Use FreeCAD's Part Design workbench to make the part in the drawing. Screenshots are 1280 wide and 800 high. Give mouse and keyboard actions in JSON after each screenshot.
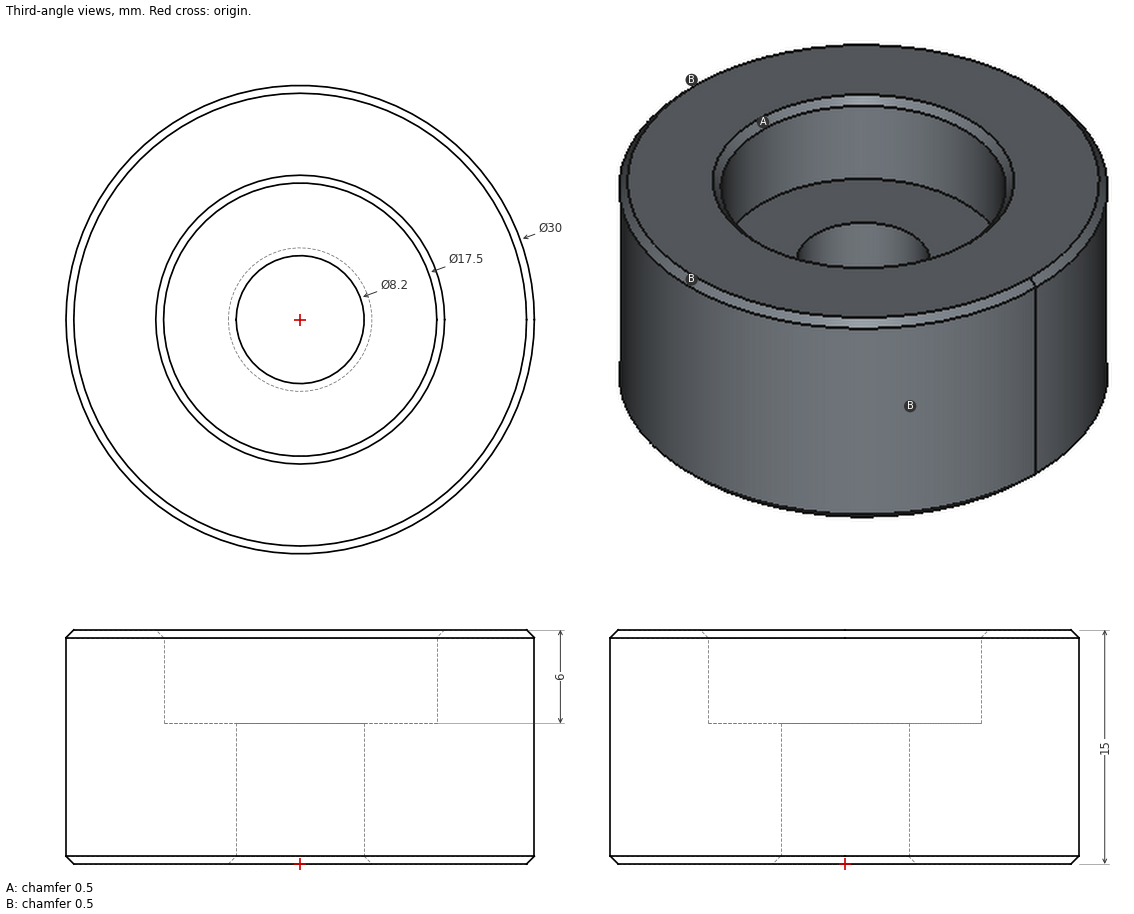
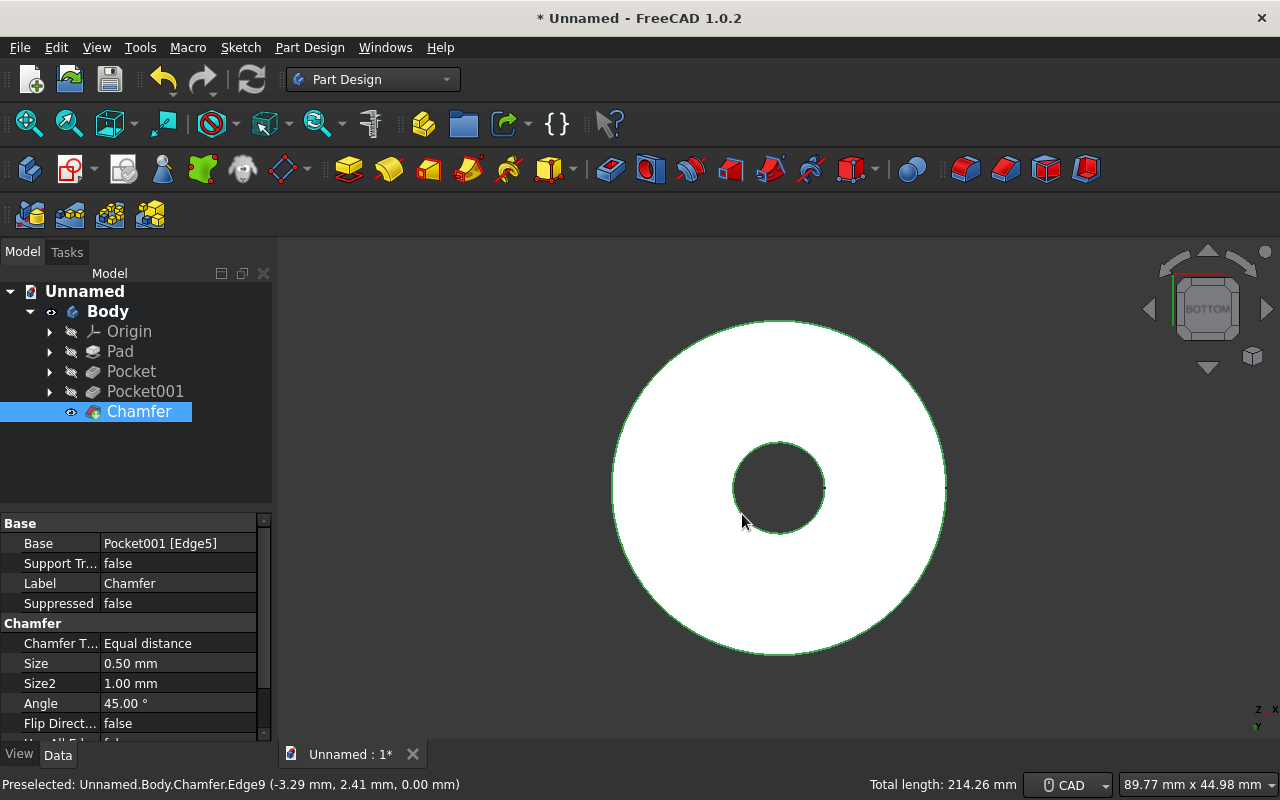
{"action": "left_click", "coordinate": [1006, 170]}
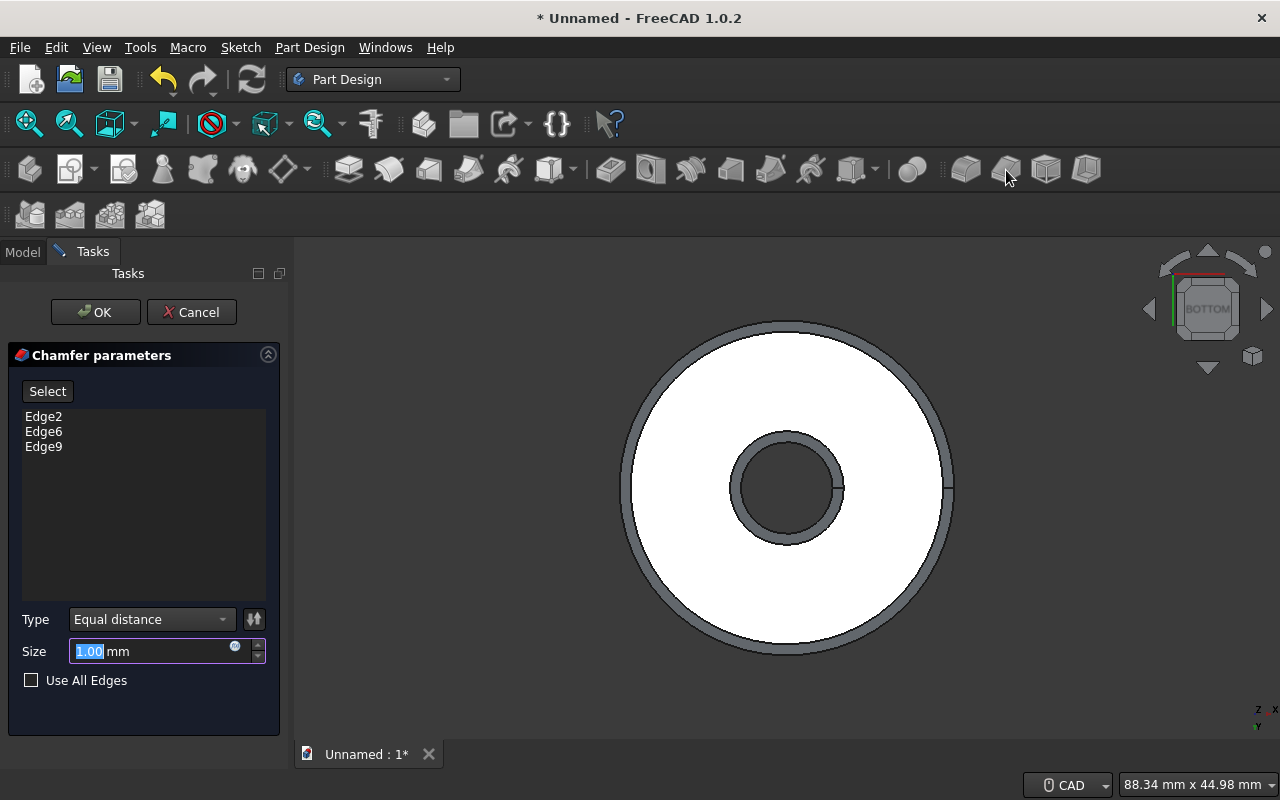
{"action": "type", "text": "0.5"}
{"action": "key", "text": "Tab"}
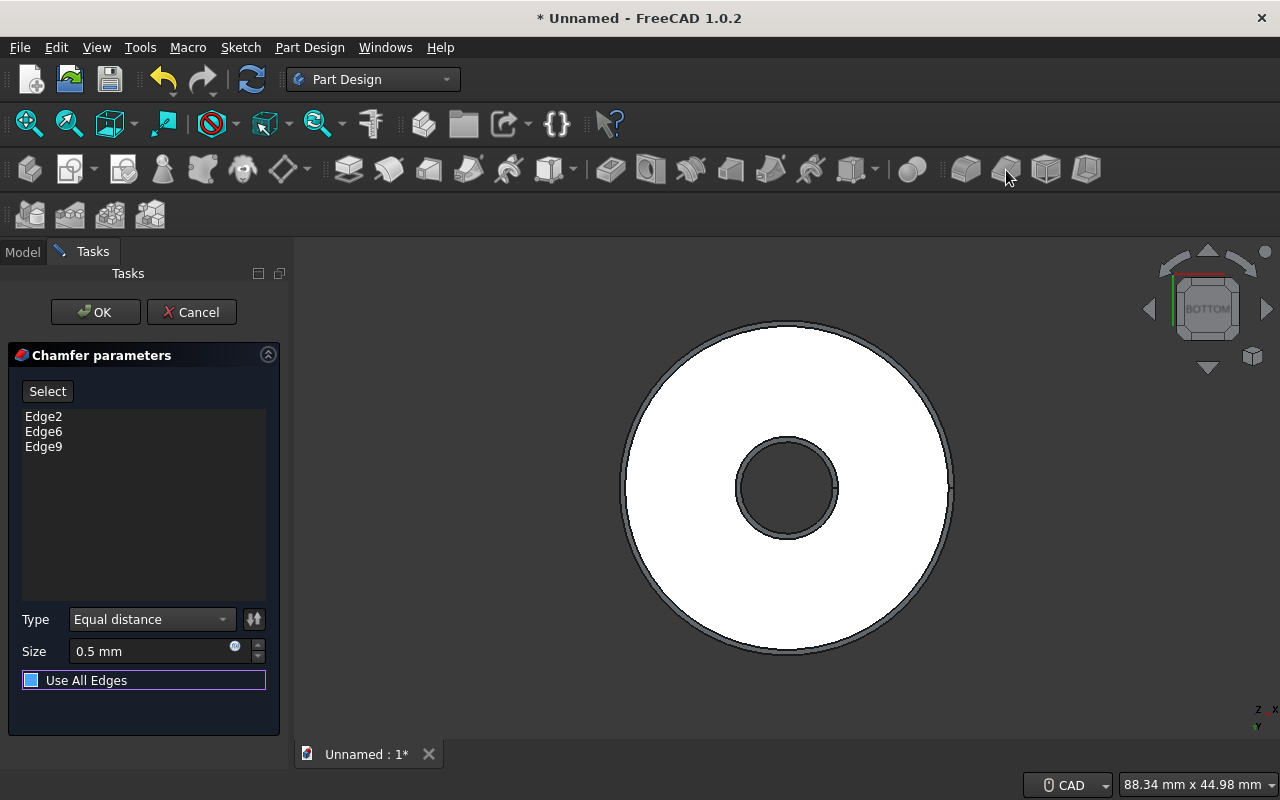
{"action": "left_click", "coordinate": [96, 312]}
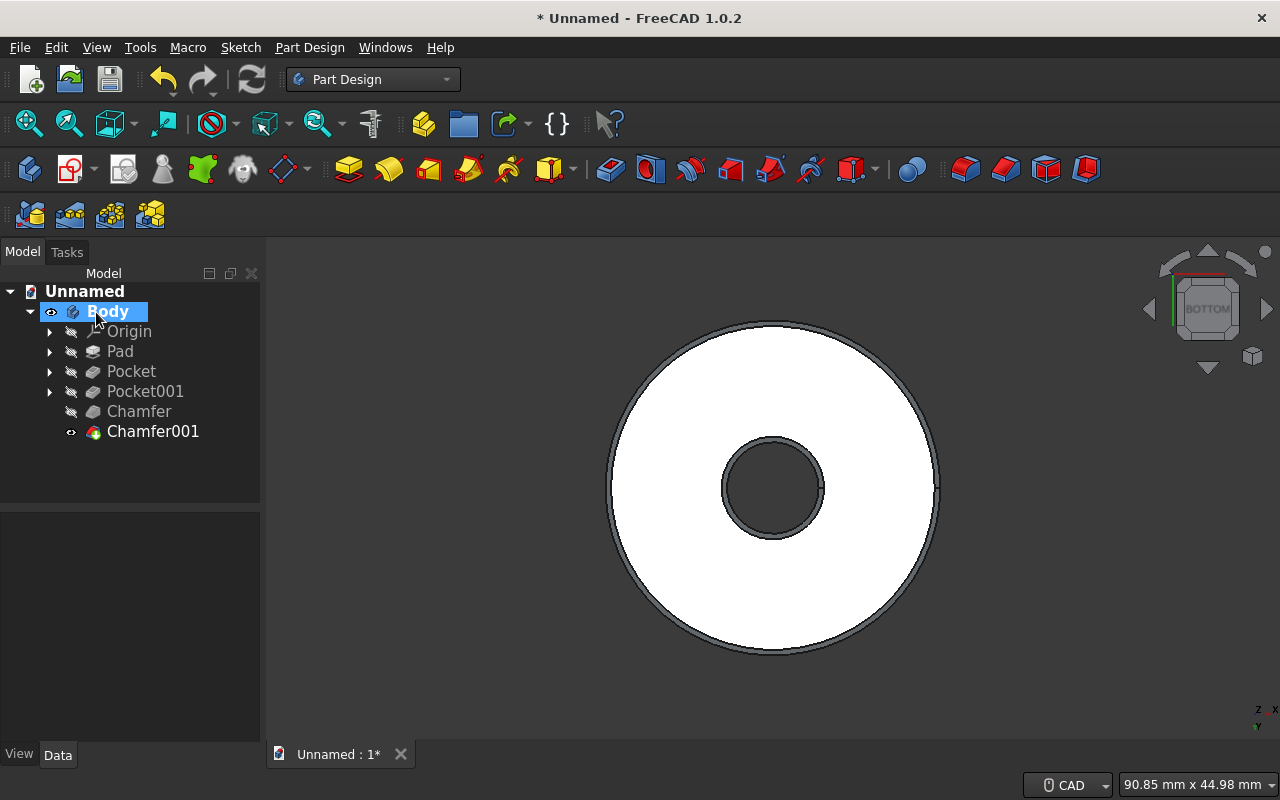
{"action": "key", "text": "0"}